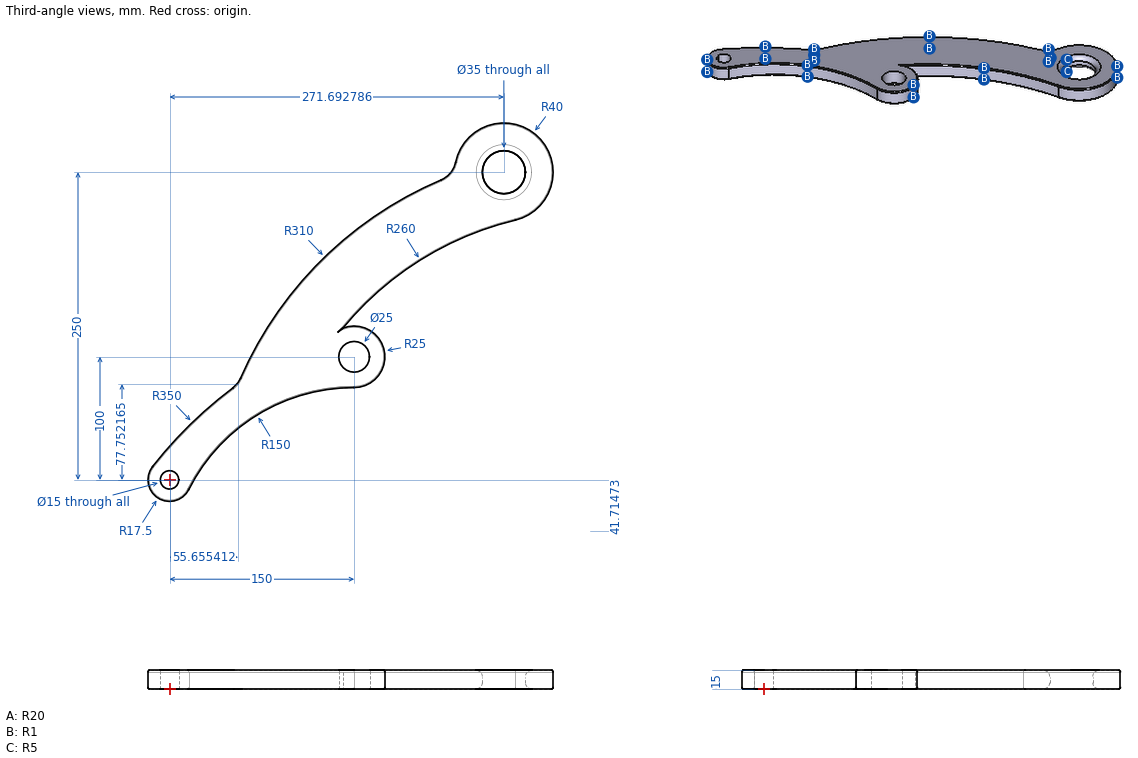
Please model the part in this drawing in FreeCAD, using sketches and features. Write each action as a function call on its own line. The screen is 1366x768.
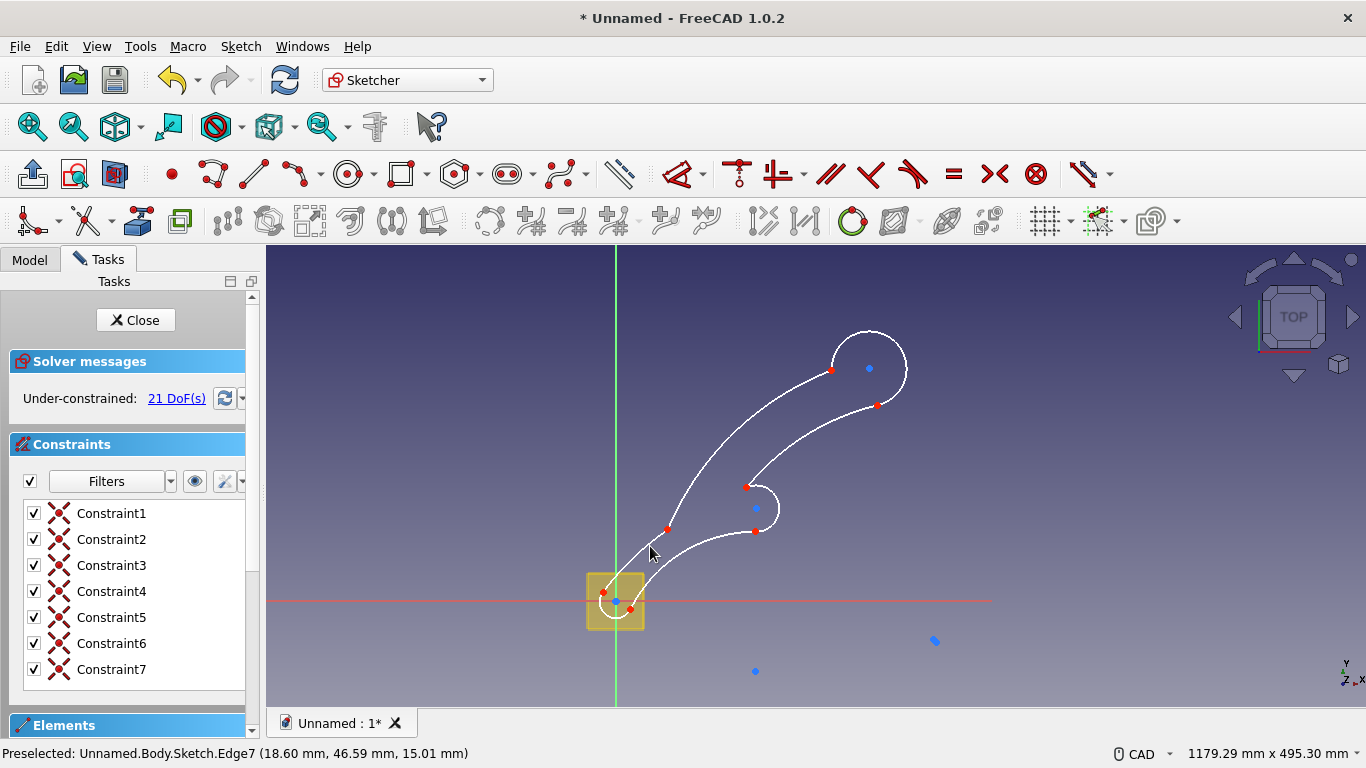
scroll(601, 608, up, 5)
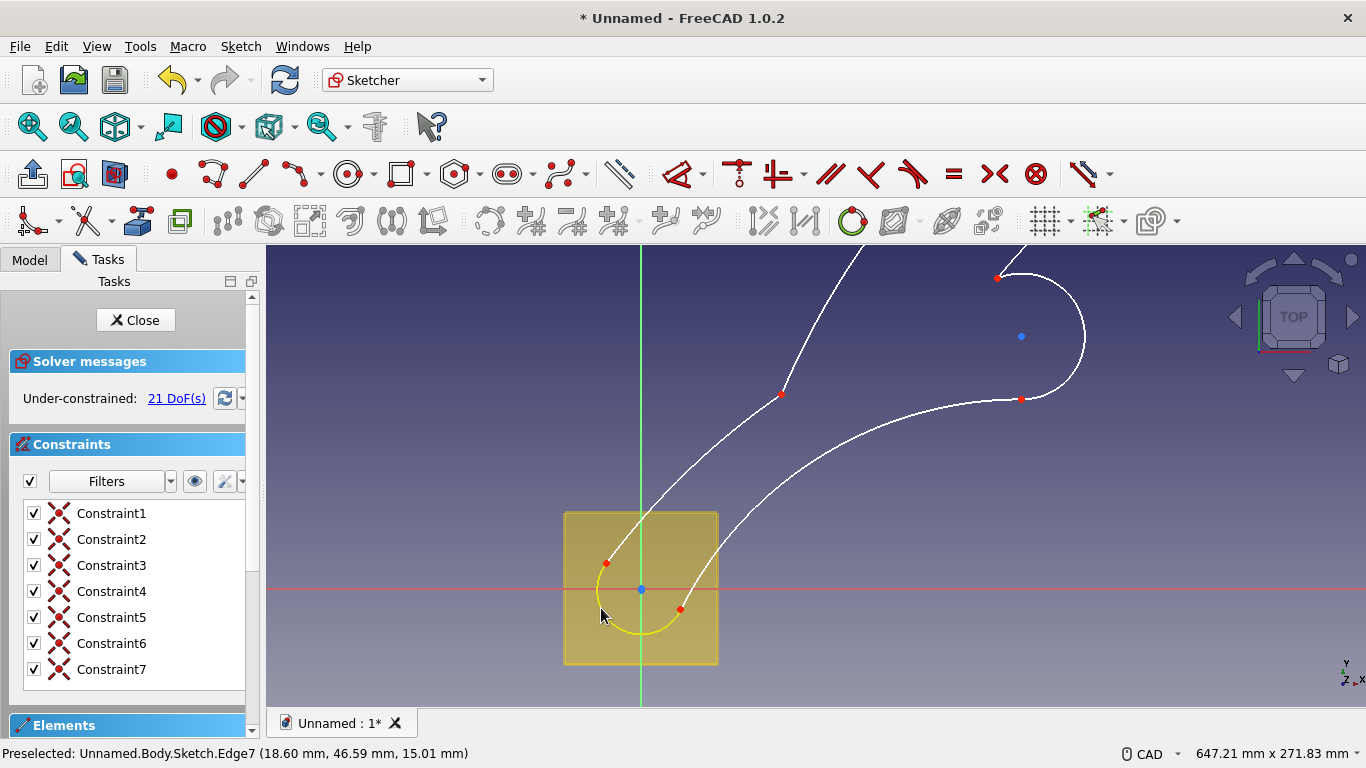
click(600, 605)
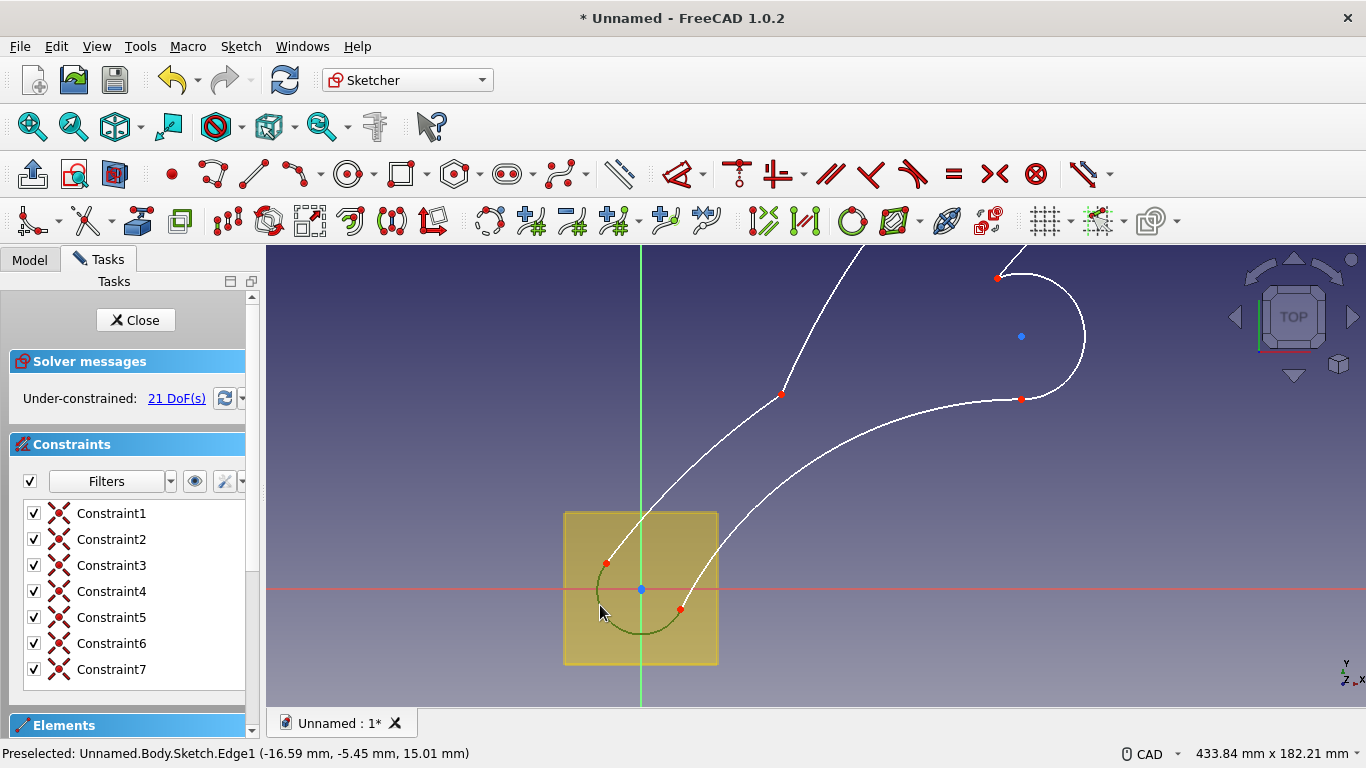
click(897, 420)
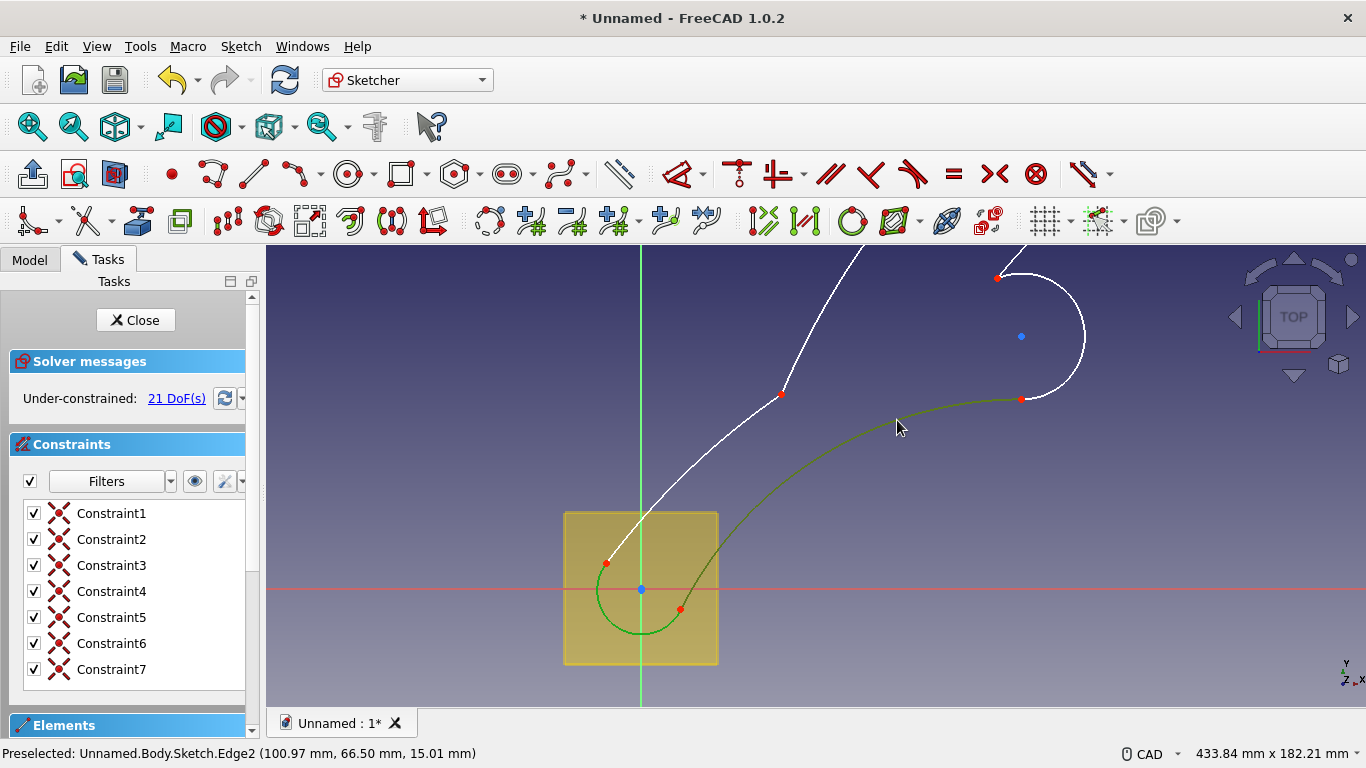
click(913, 174)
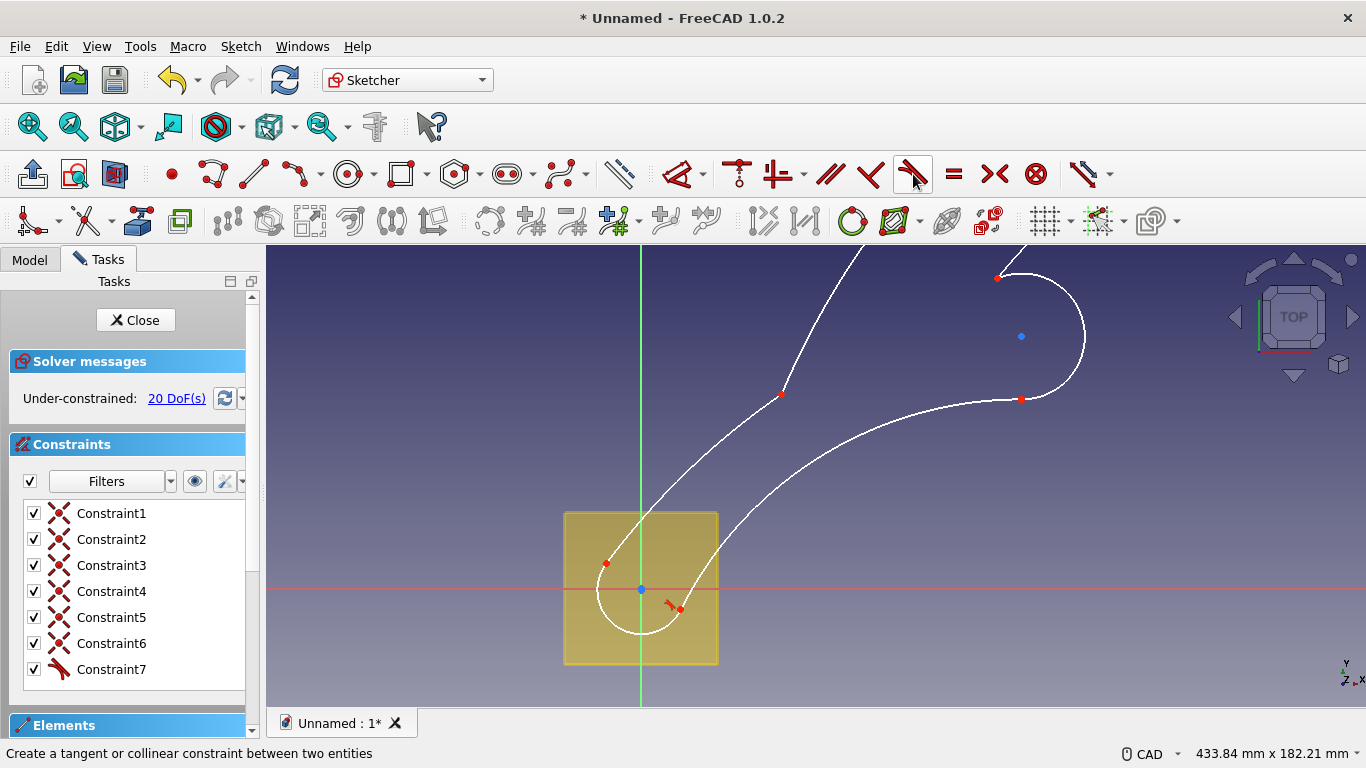
click(600, 605)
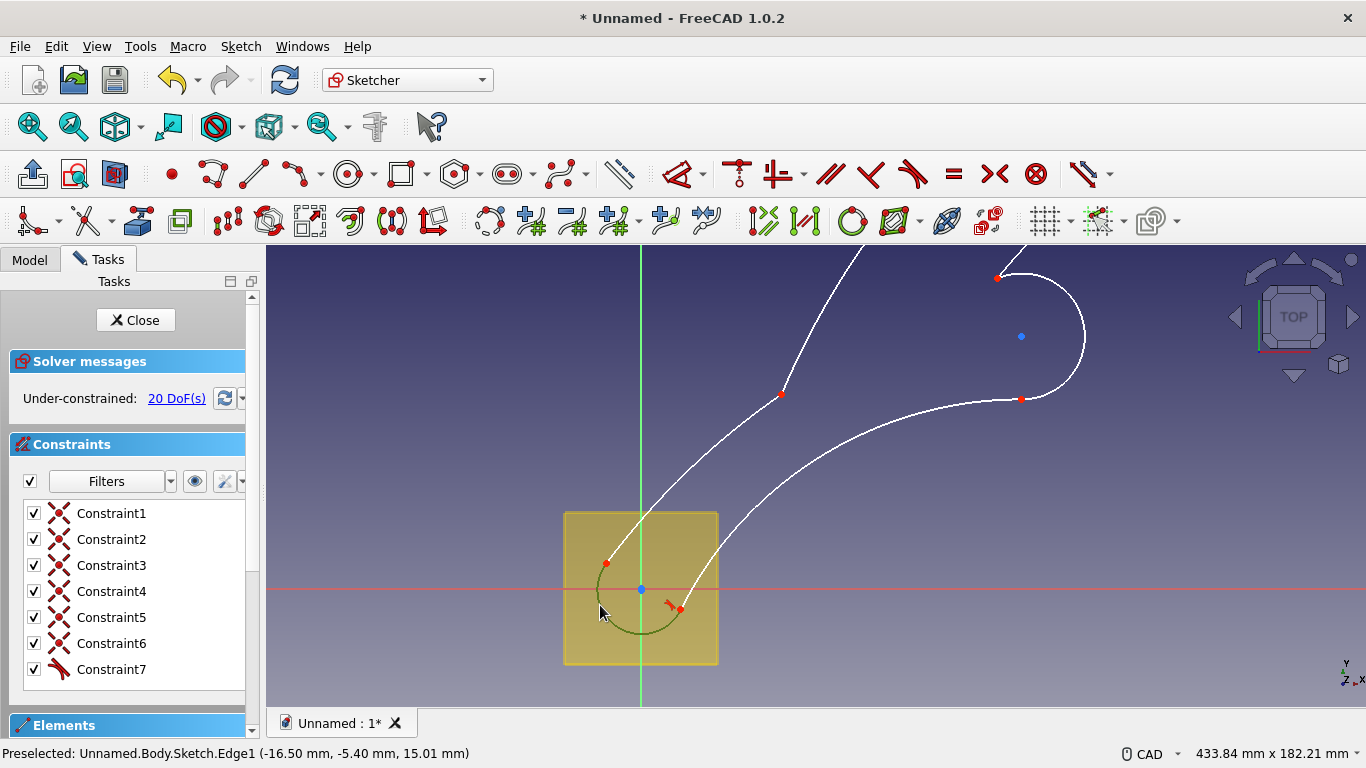
click(723, 439)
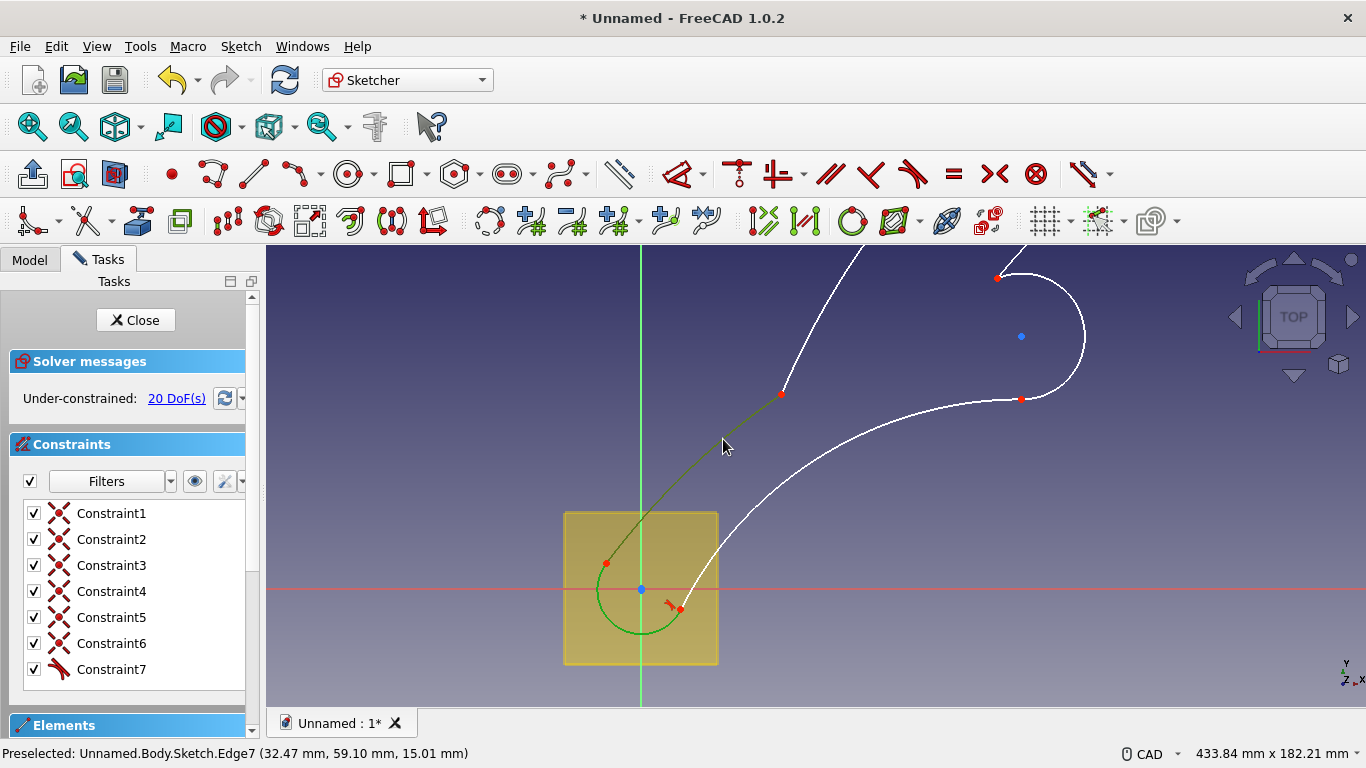
key(t)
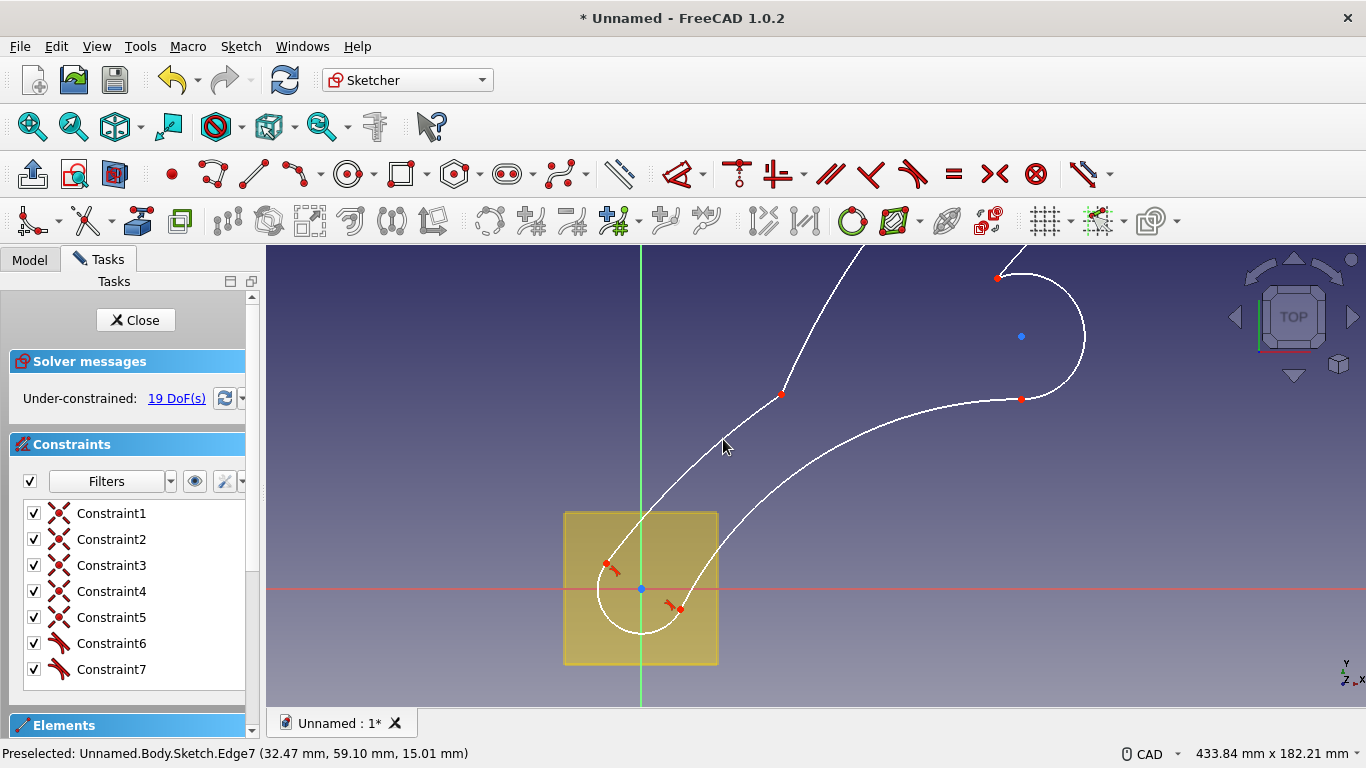
click(897, 420)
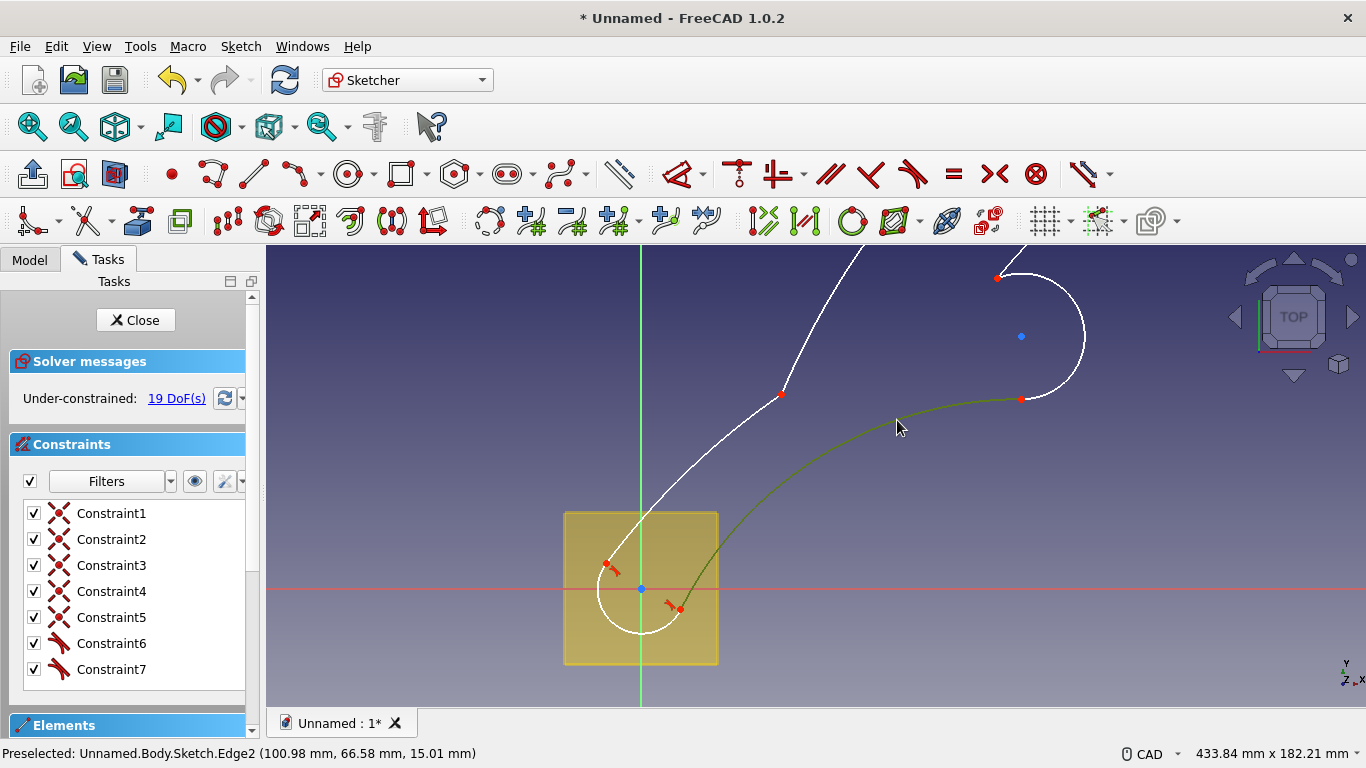
click(1077, 367)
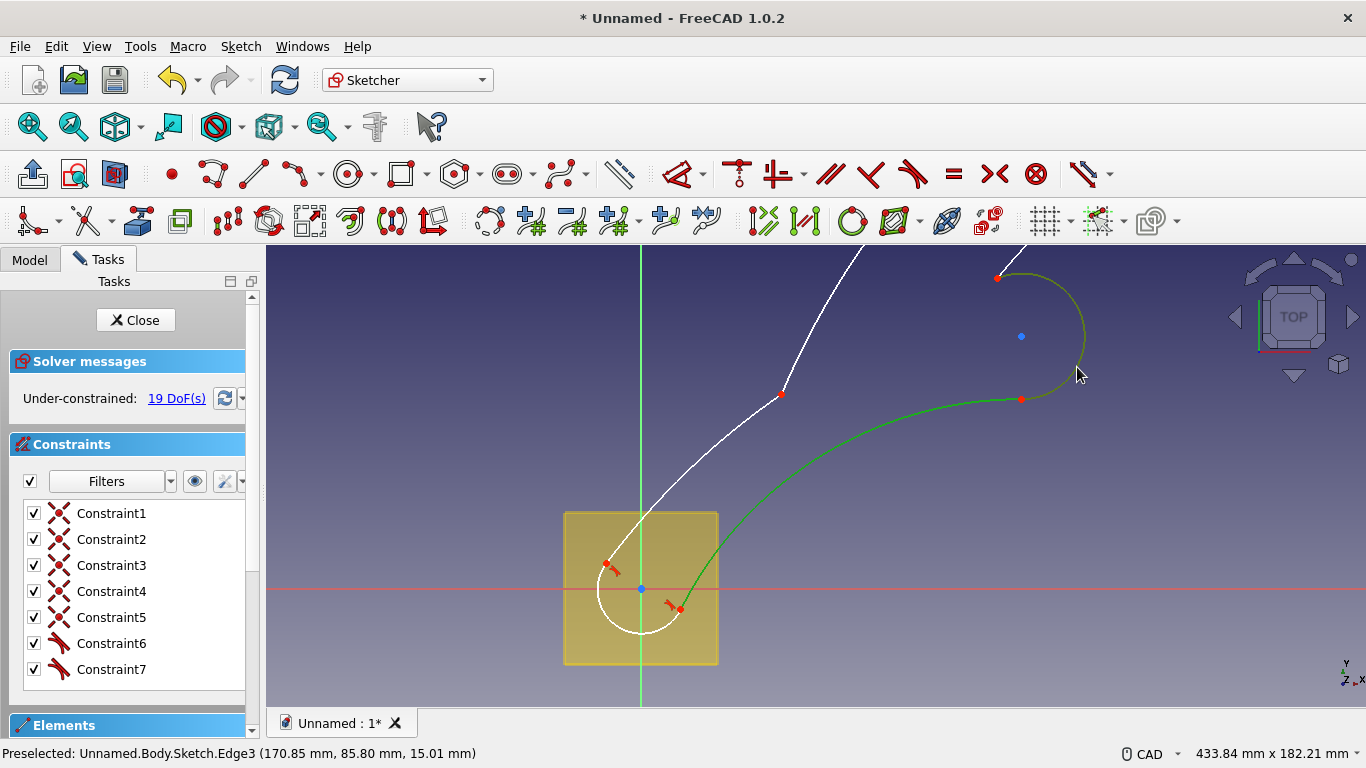
click(913, 174)